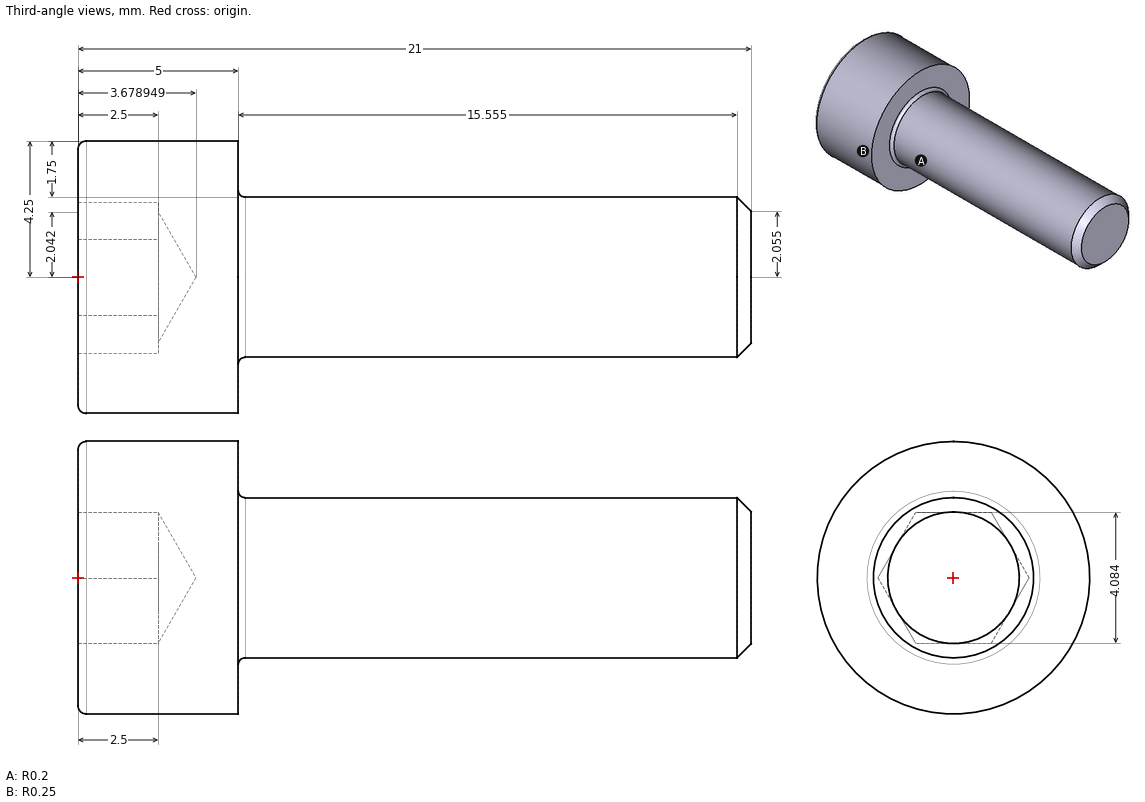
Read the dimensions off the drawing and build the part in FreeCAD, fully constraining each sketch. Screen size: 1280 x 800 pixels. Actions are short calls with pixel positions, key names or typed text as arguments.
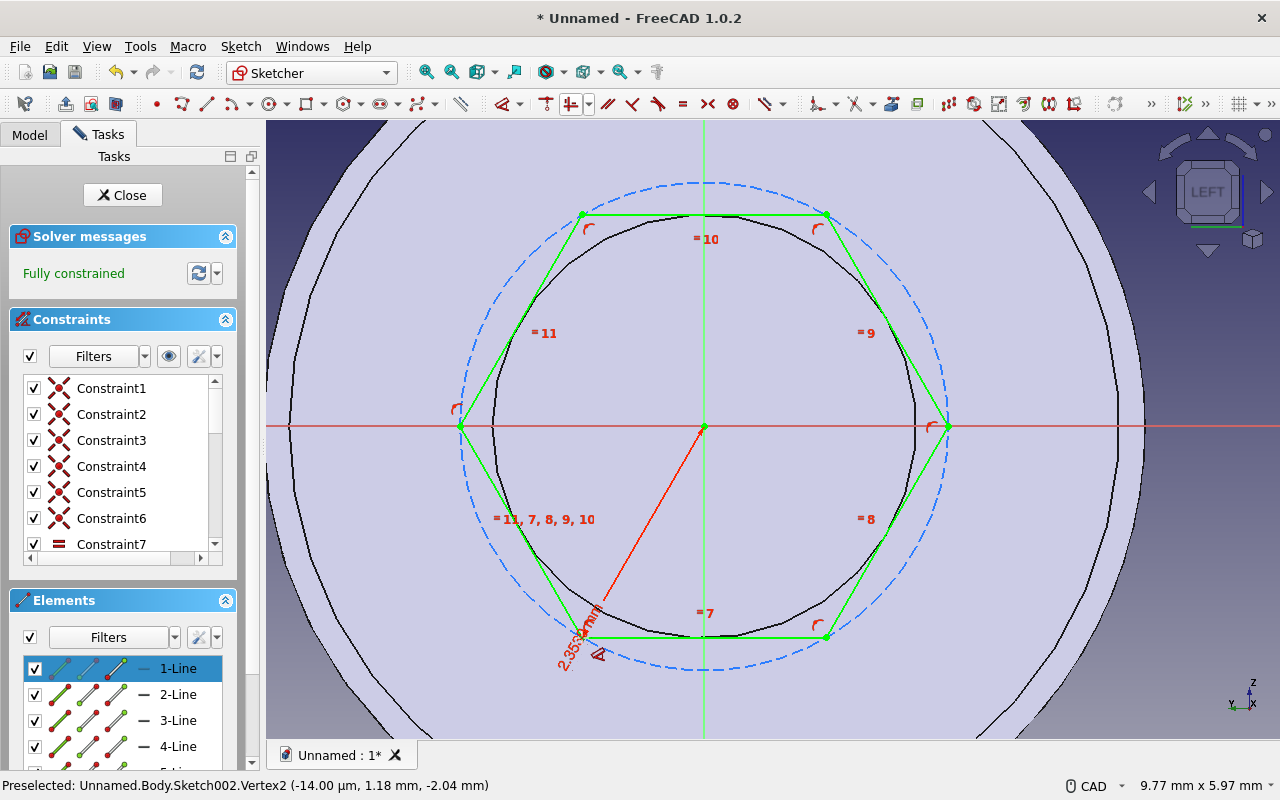
click(826, 215)
click(860, 329)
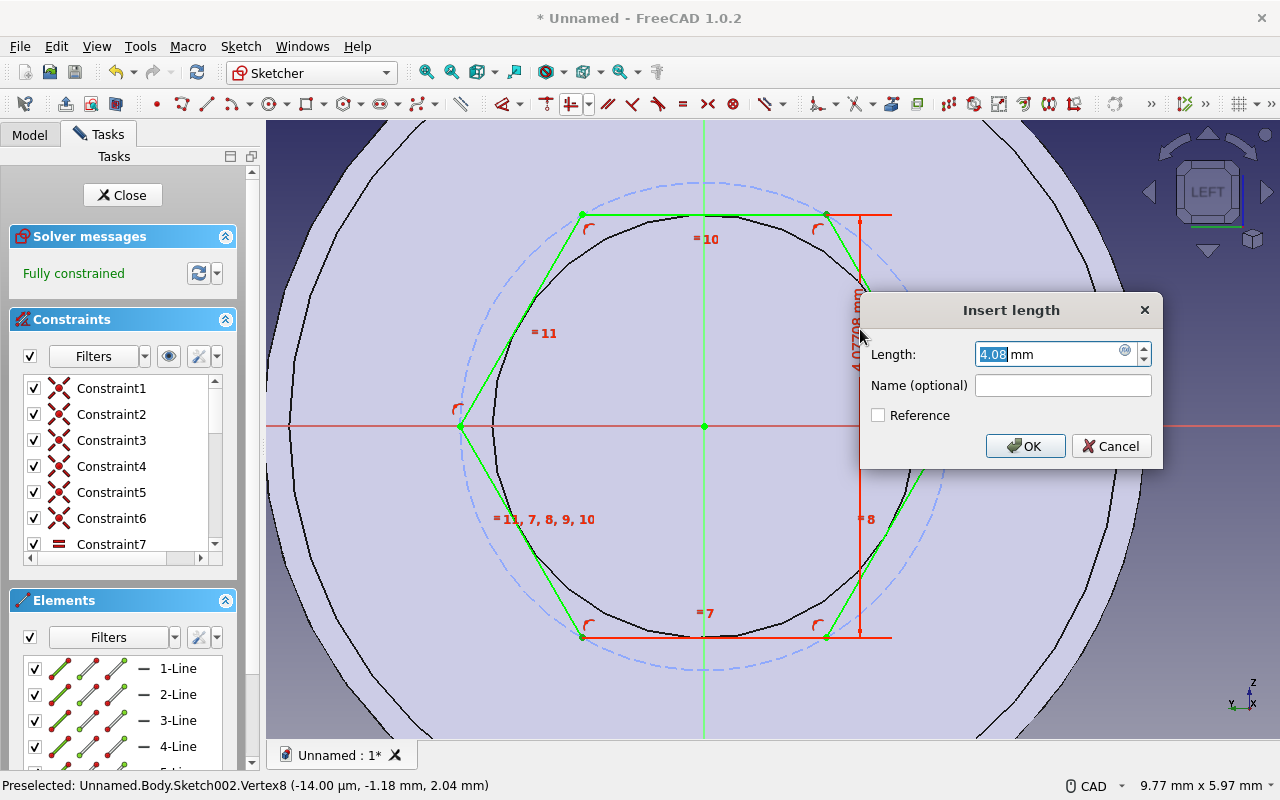
text(4.084)
key(Return)
key(Escape)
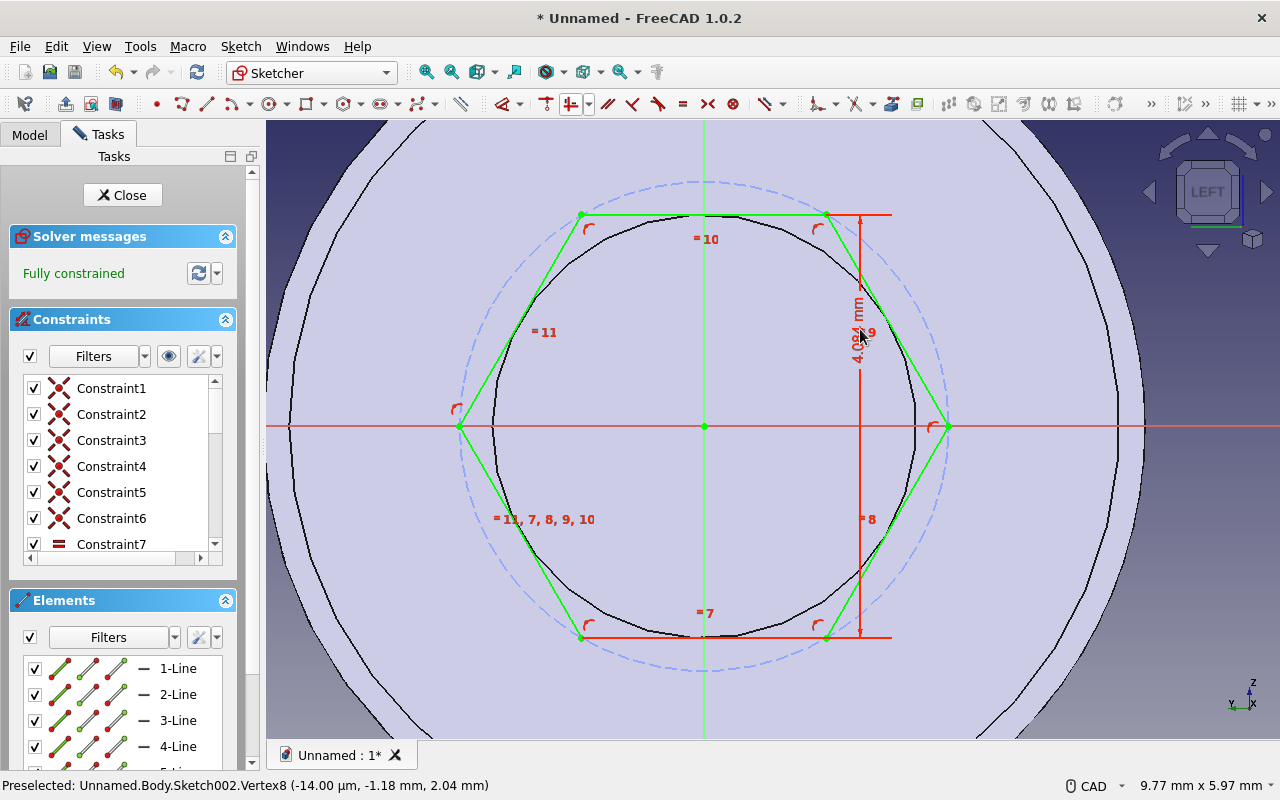
click(123, 195)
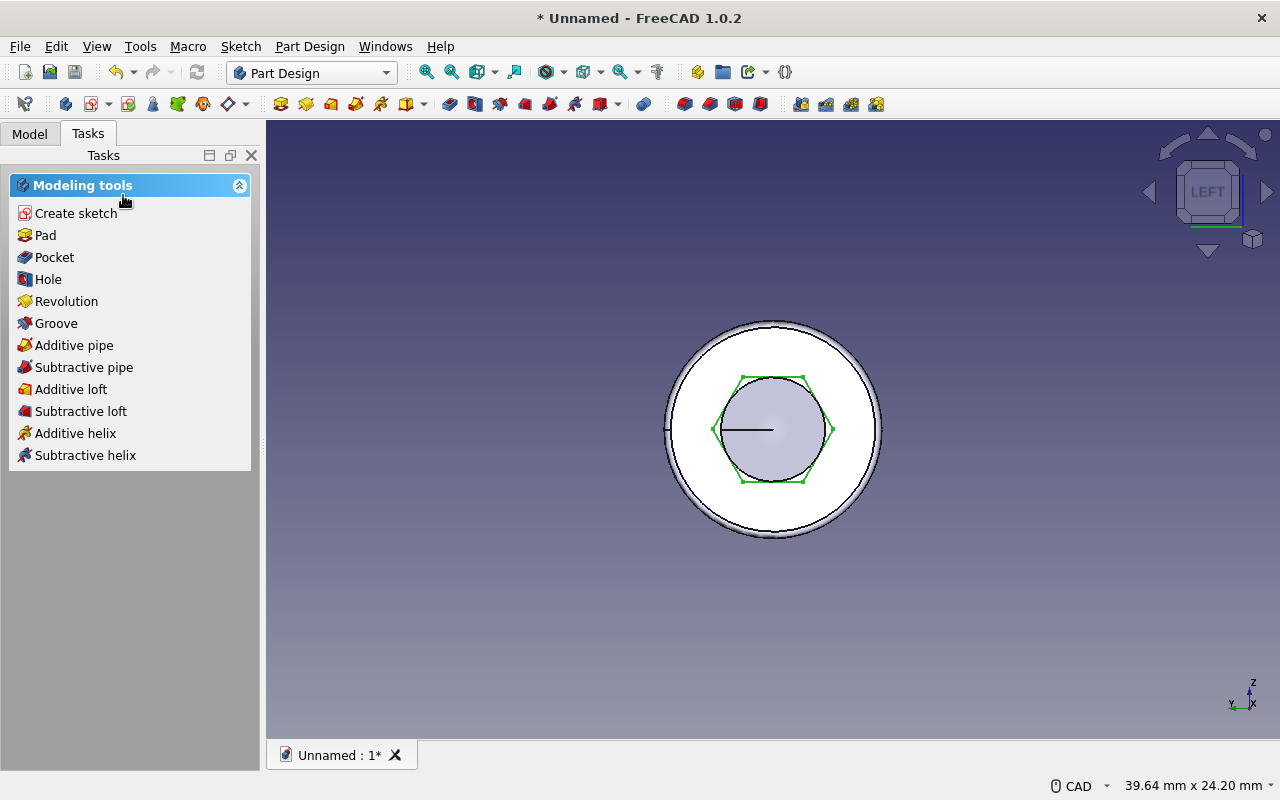
click(450, 104)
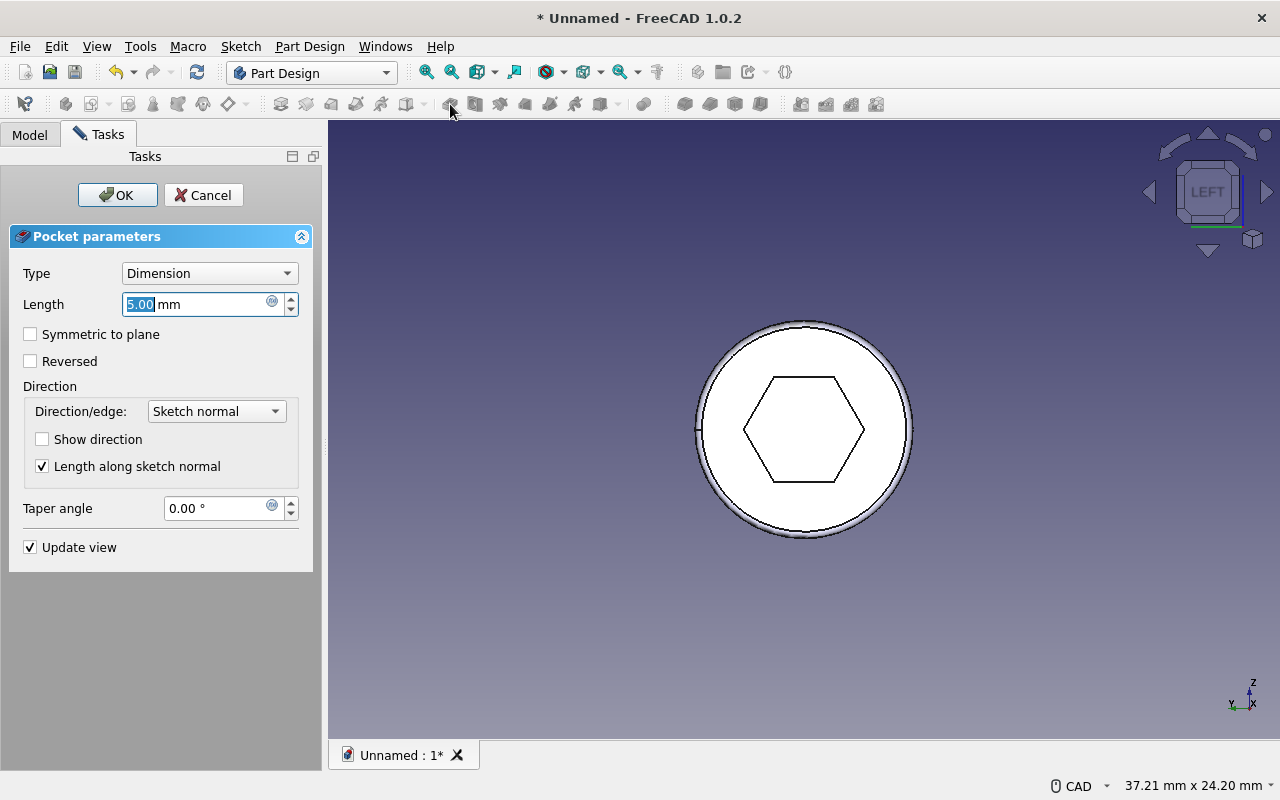
text(2.5)
key(Tab)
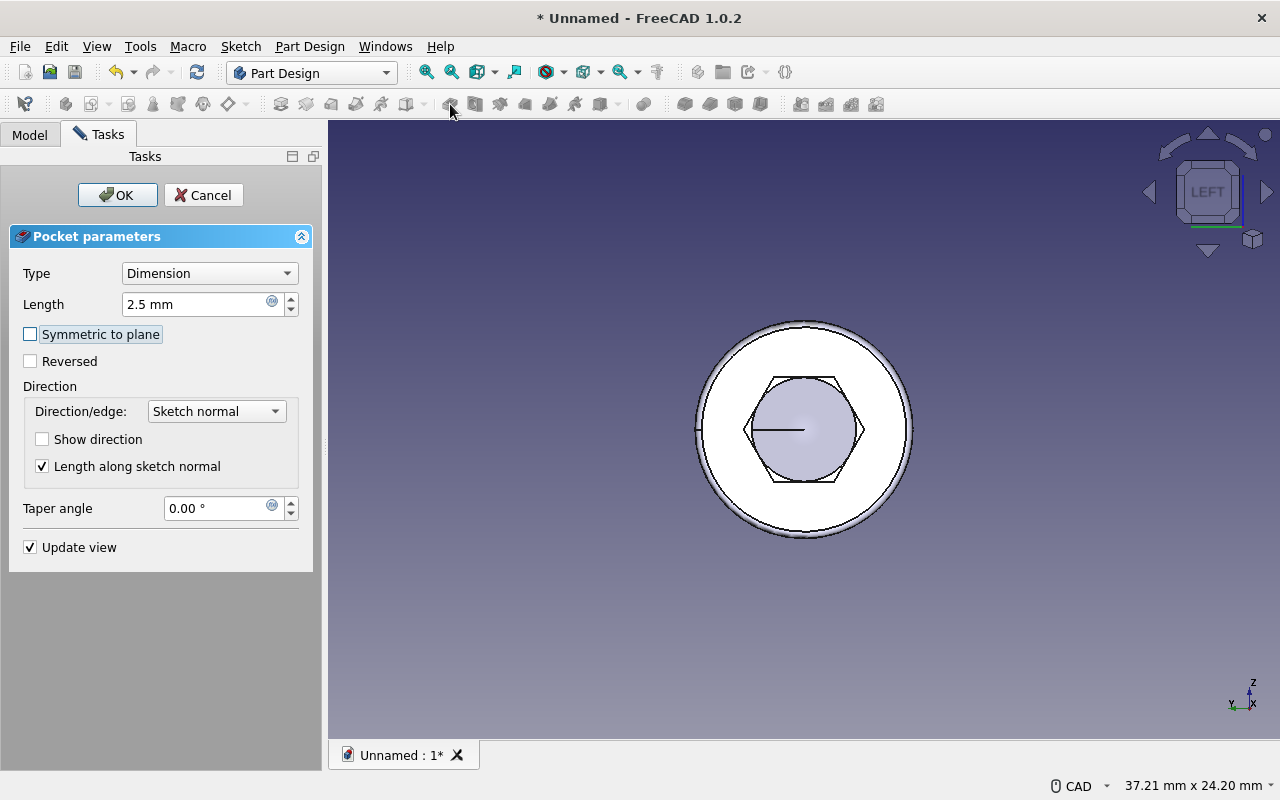
click(118, 195)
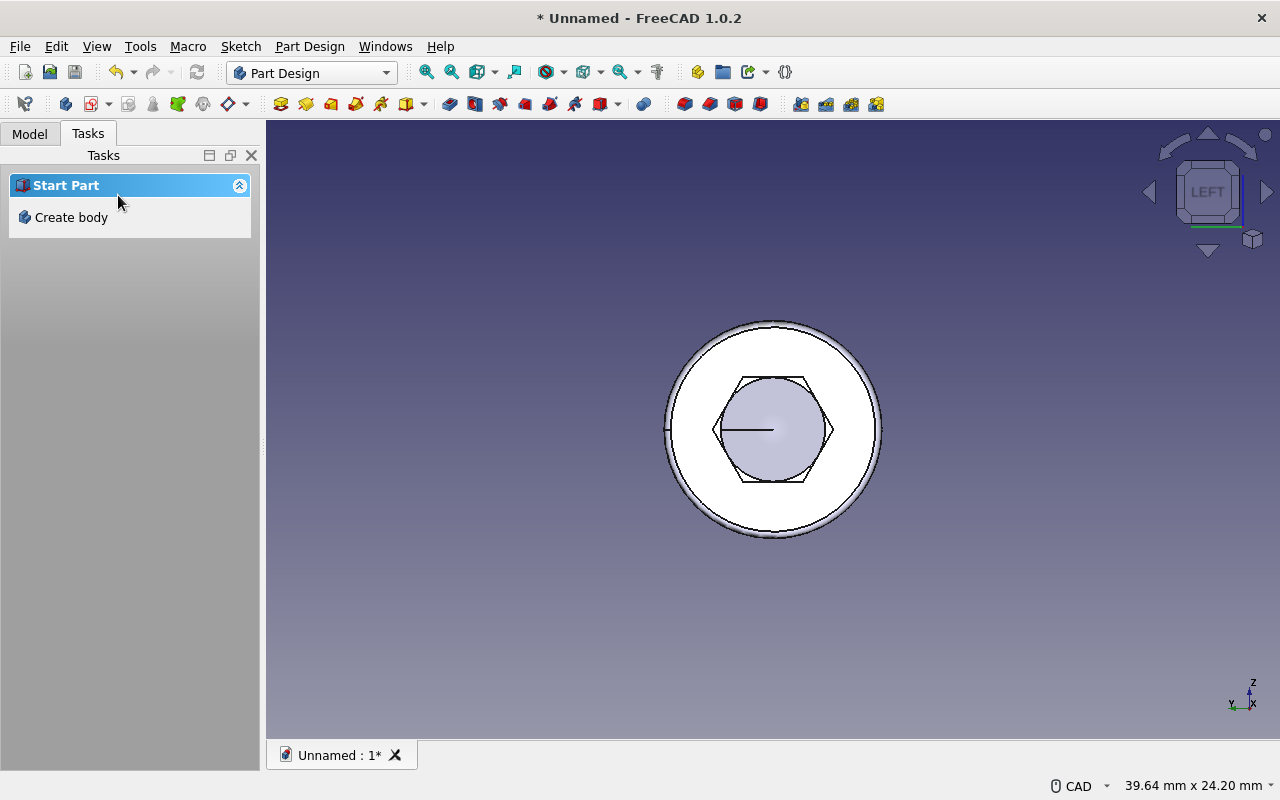
key(0)